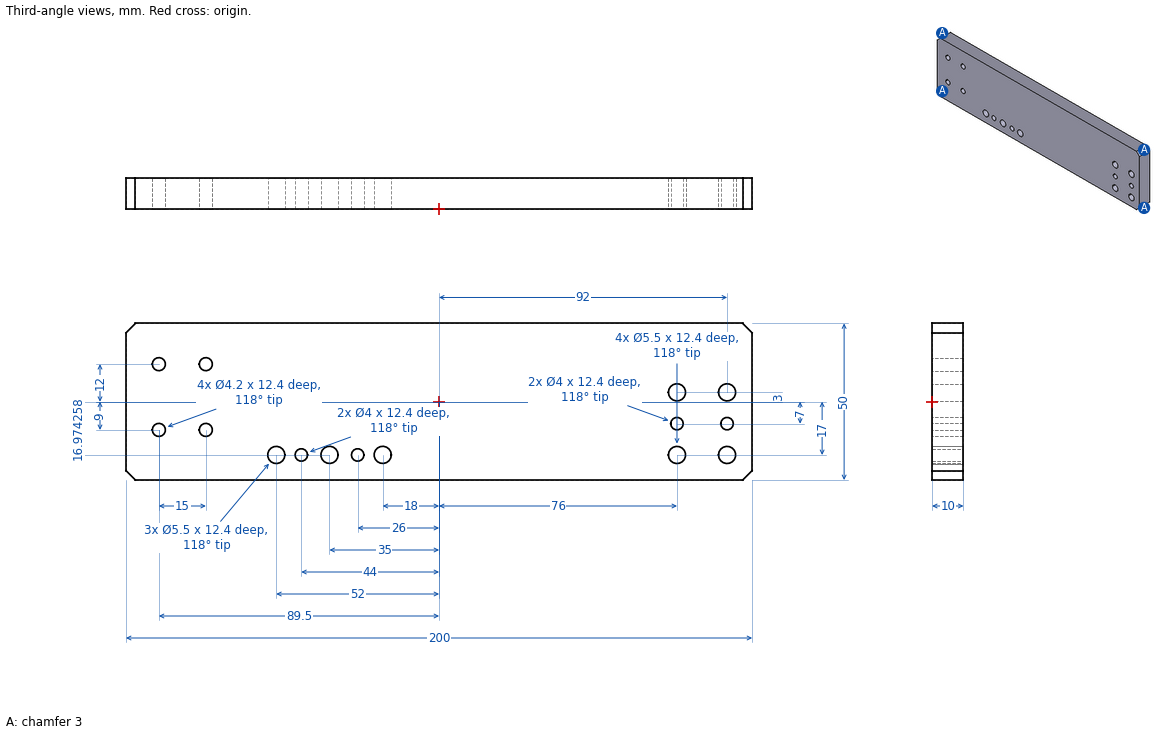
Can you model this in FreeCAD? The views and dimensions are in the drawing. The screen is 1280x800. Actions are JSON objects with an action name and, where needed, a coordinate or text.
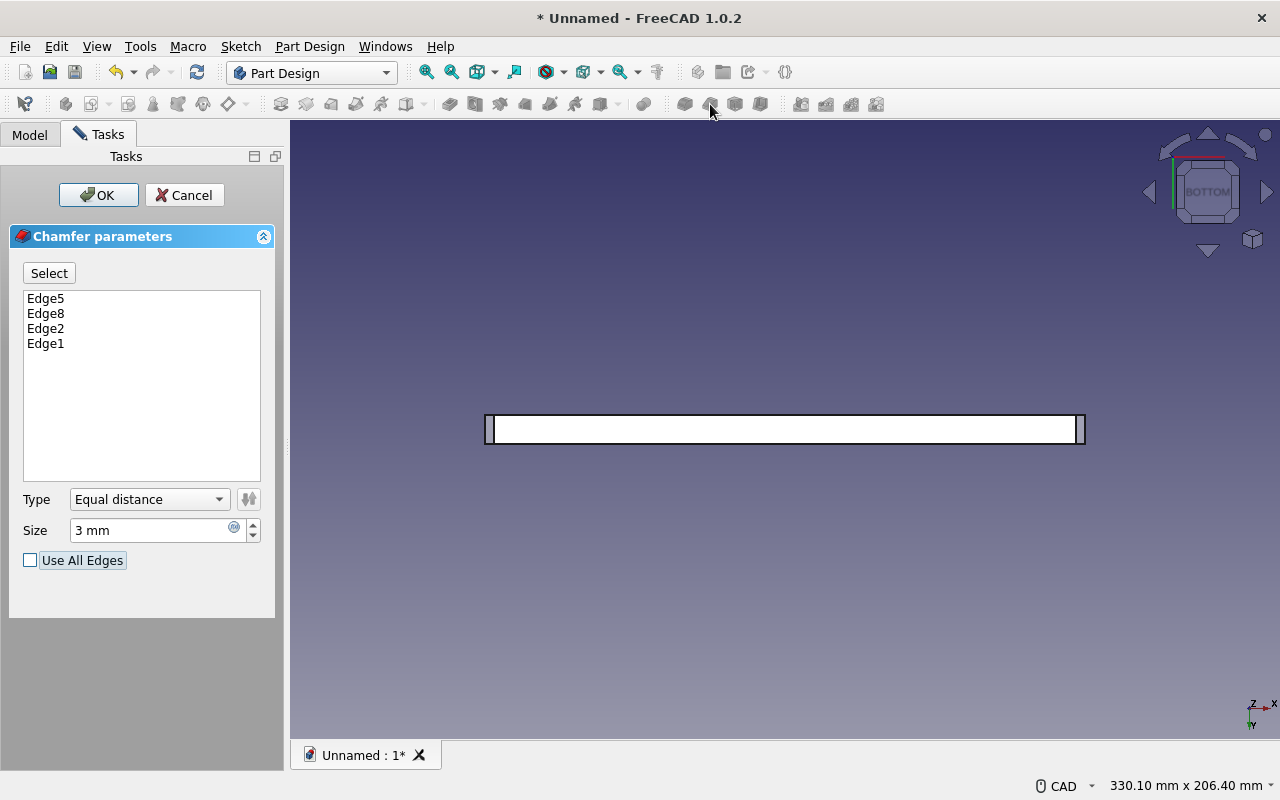
{"action": "left_click", "coordinate": [99, 195]}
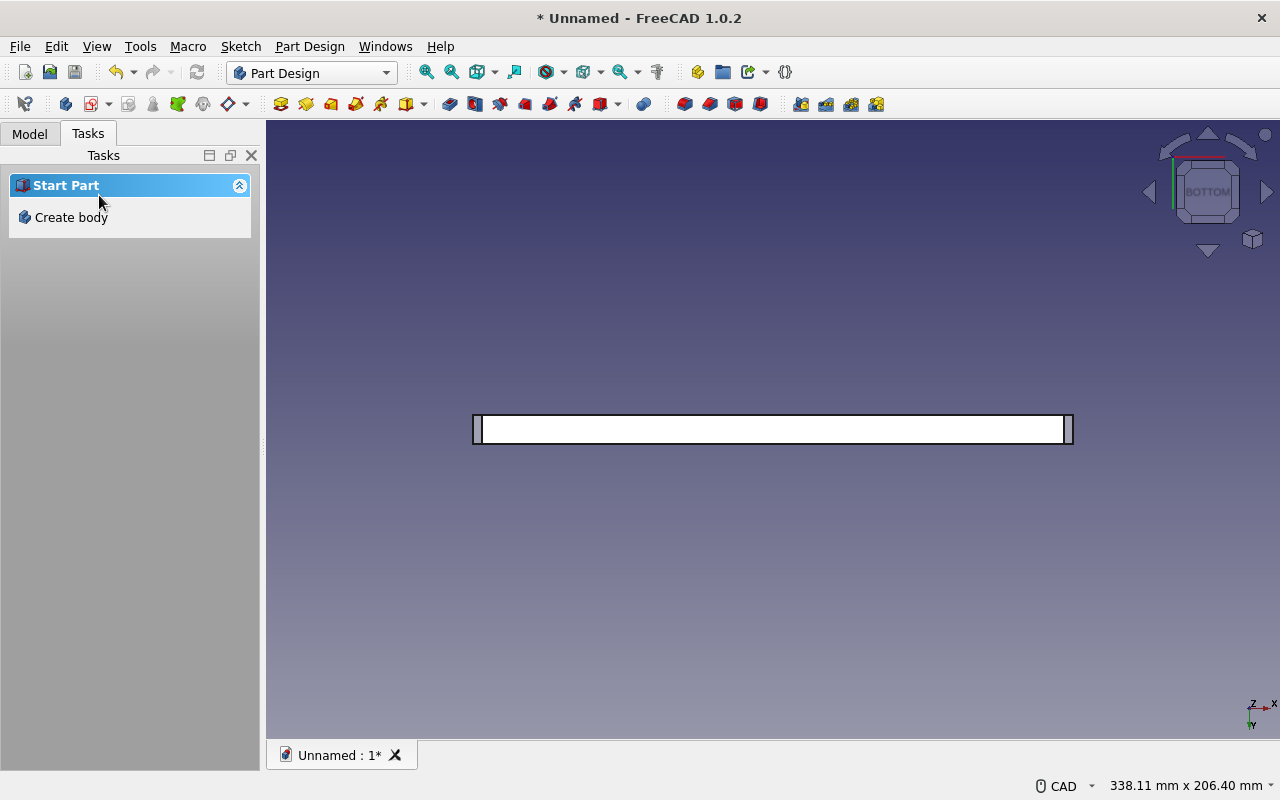
{"action": "key", "text": "4"}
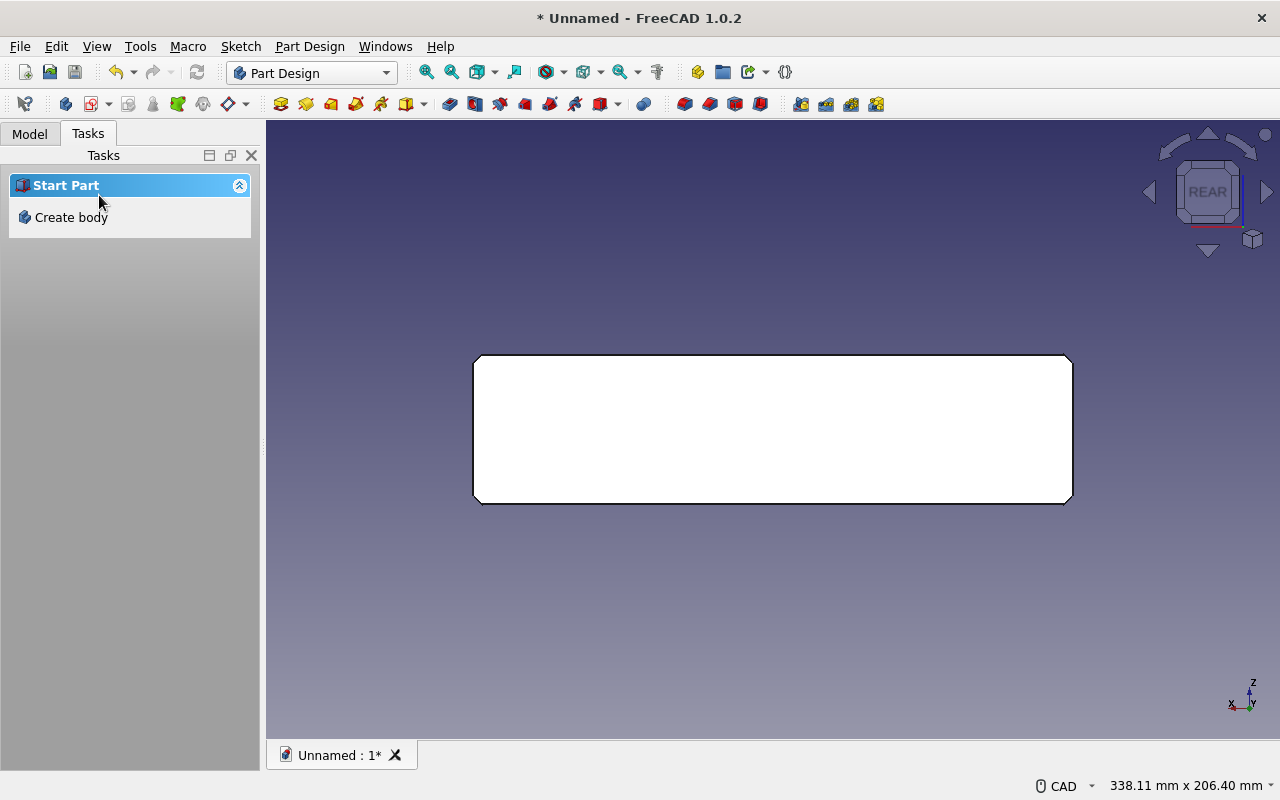
{"action": "left_click", "coordinate": [602, 429]}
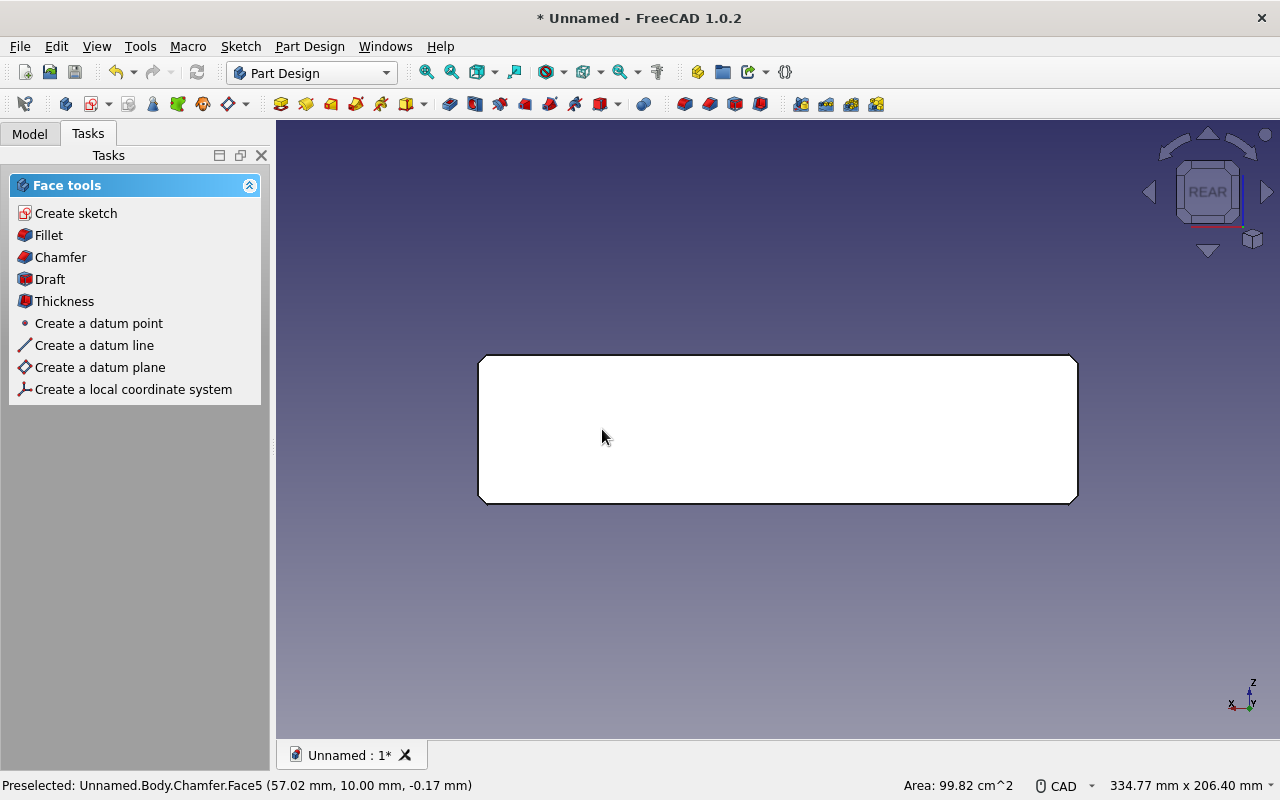
{"action": "left_click", "coordinate": [90, 104]}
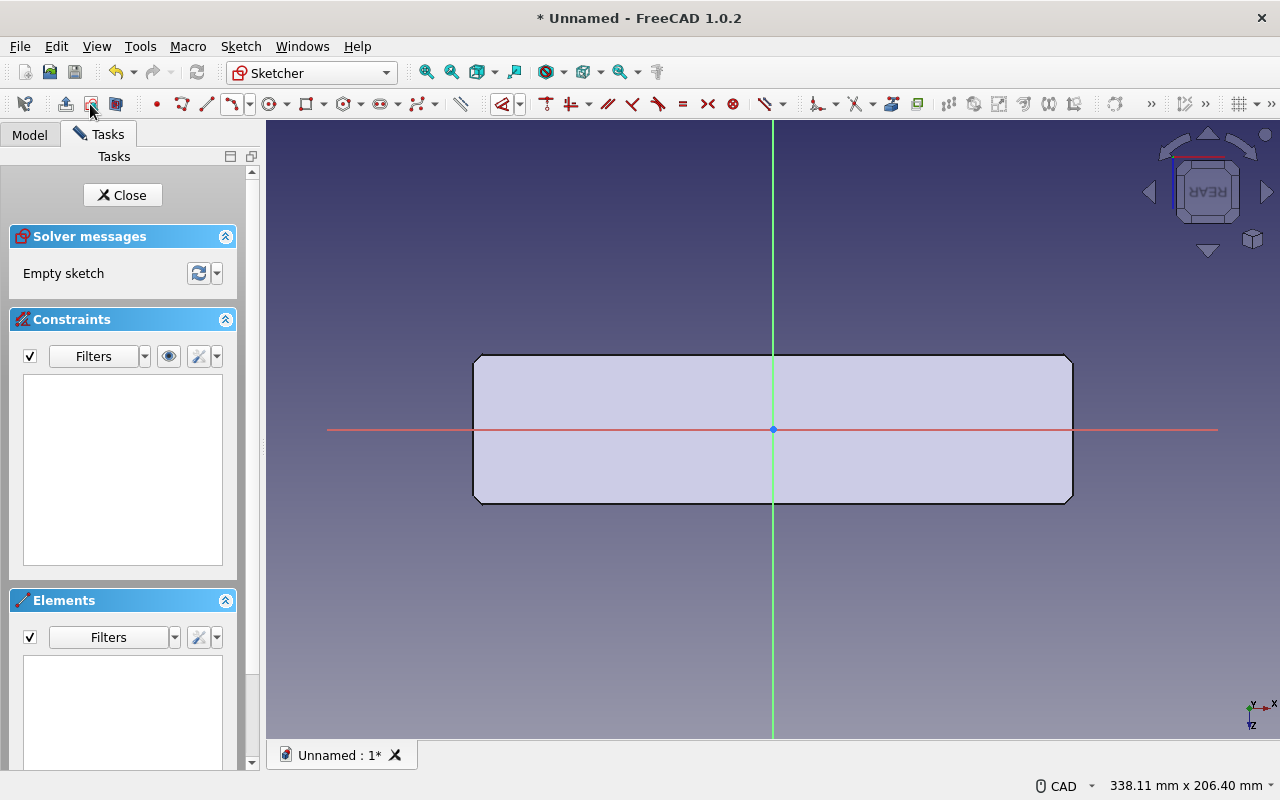
{"action": "scroll", "coordinate": [1106, 403], "scroll_direction": "up", "scroll_amount": 8}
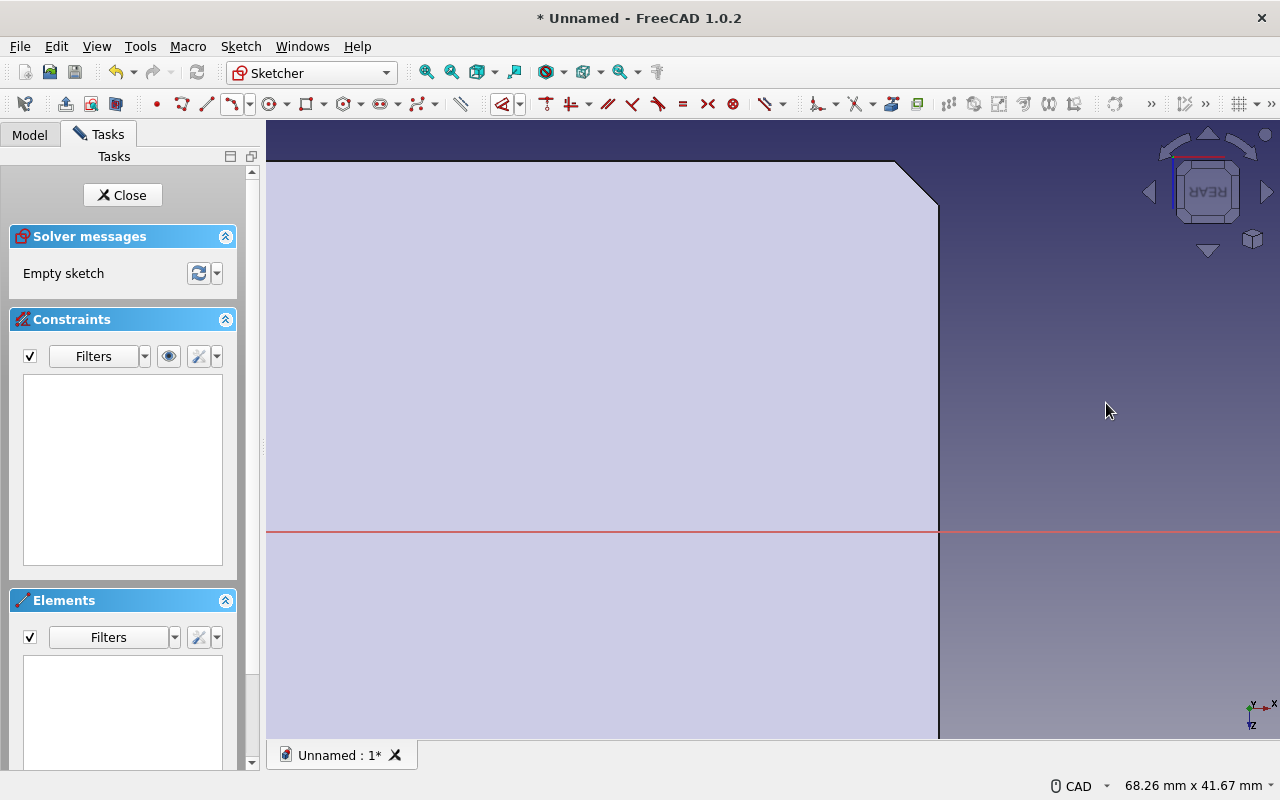
{"action": "key", "text": "g c"}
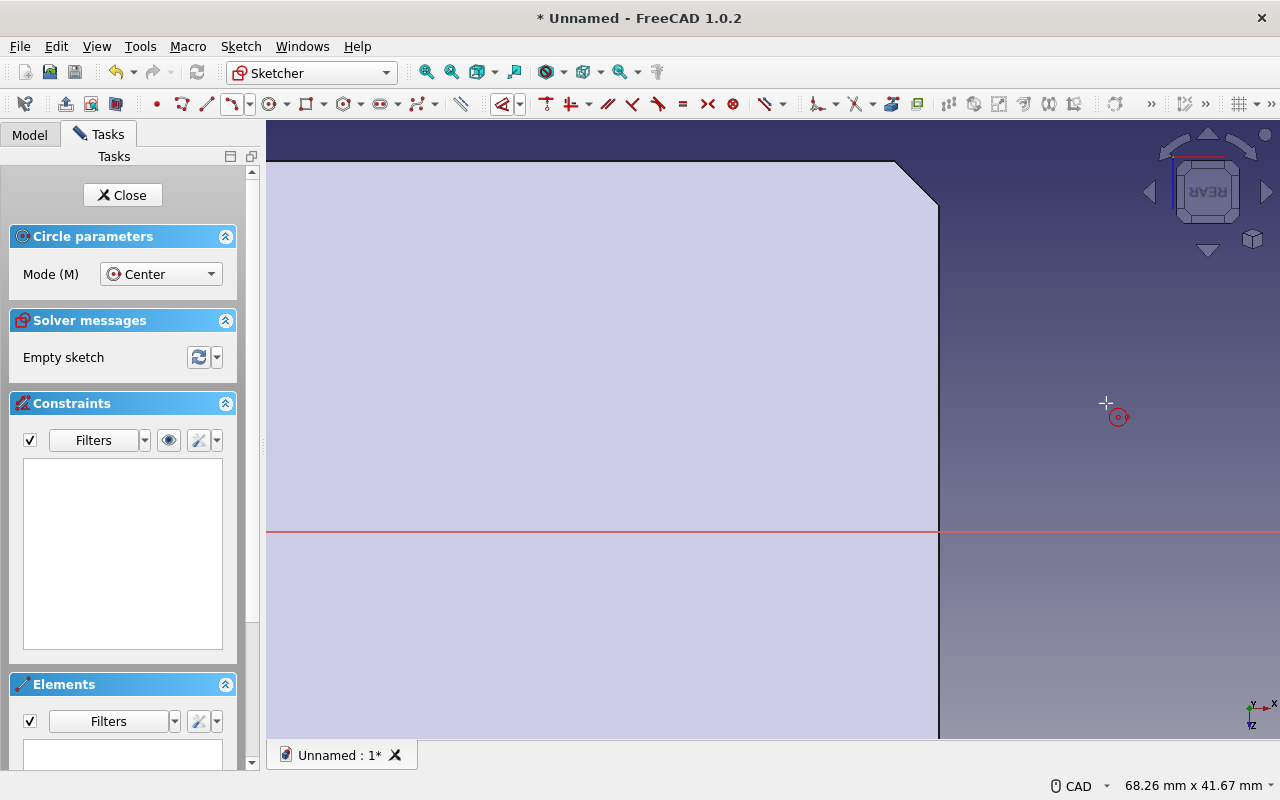
{"action": "left_click", "coordinate": [582, 280]}
{"action": "left_click", "coordinate": [611, 251]}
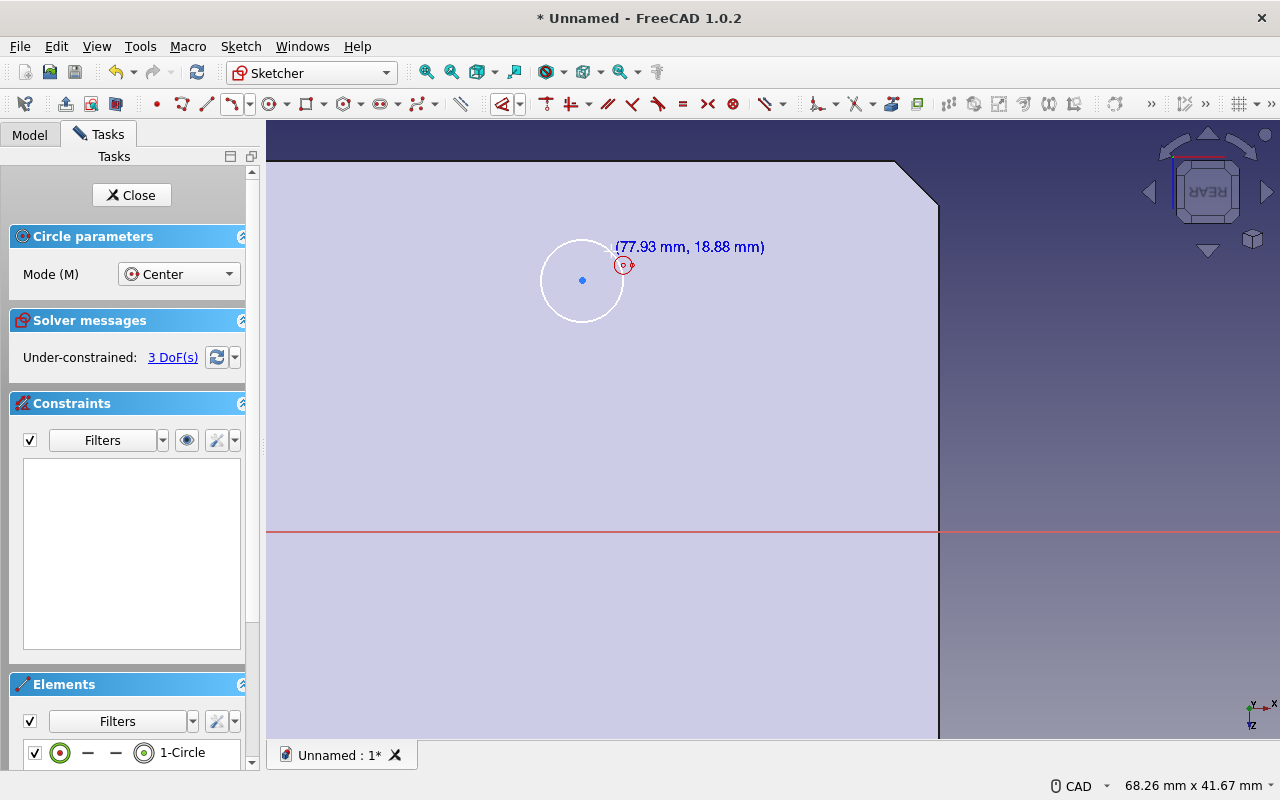
{"action": "left_click", "coordinate": [582, 577]}
{"action": "left_click", "coordinate": [611, 548]}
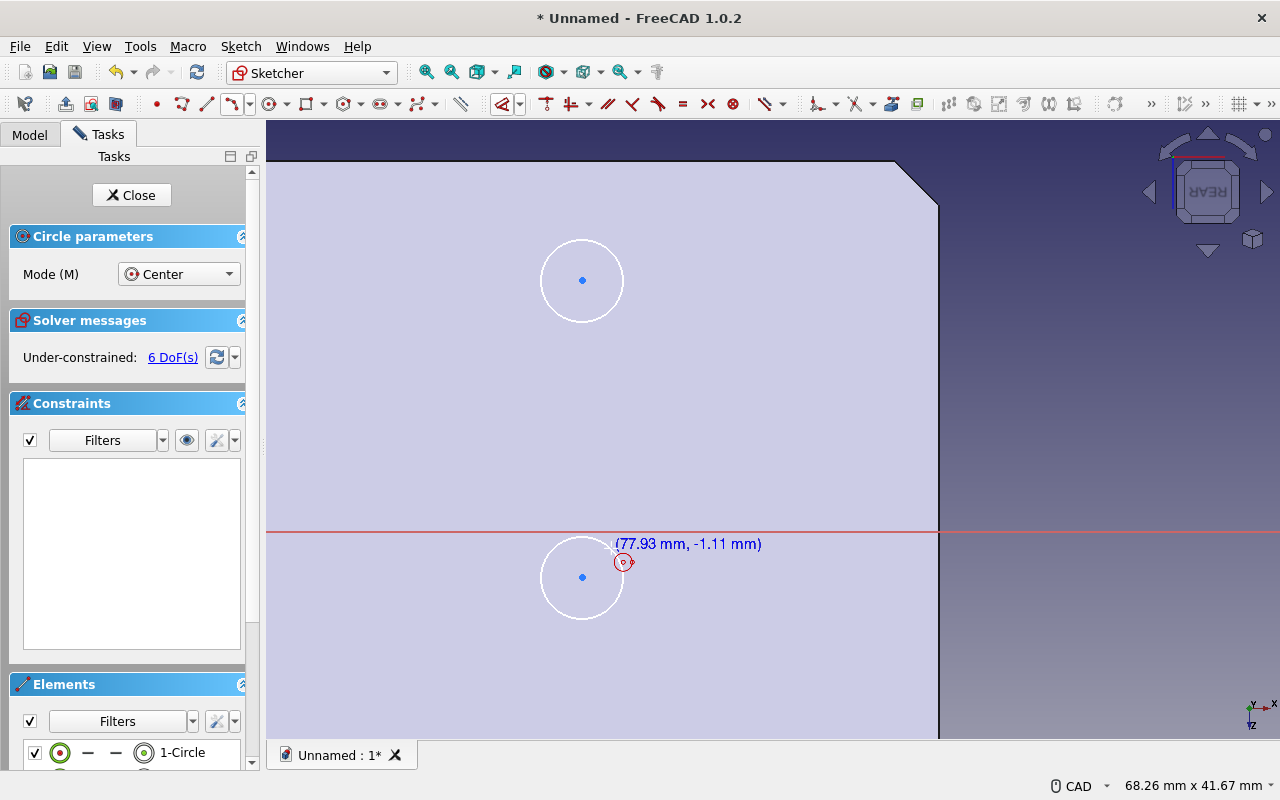
{"action": "left_click", "coordinate": [820, 577]}
{"action": "left_click", "coordinate": [849, 548]}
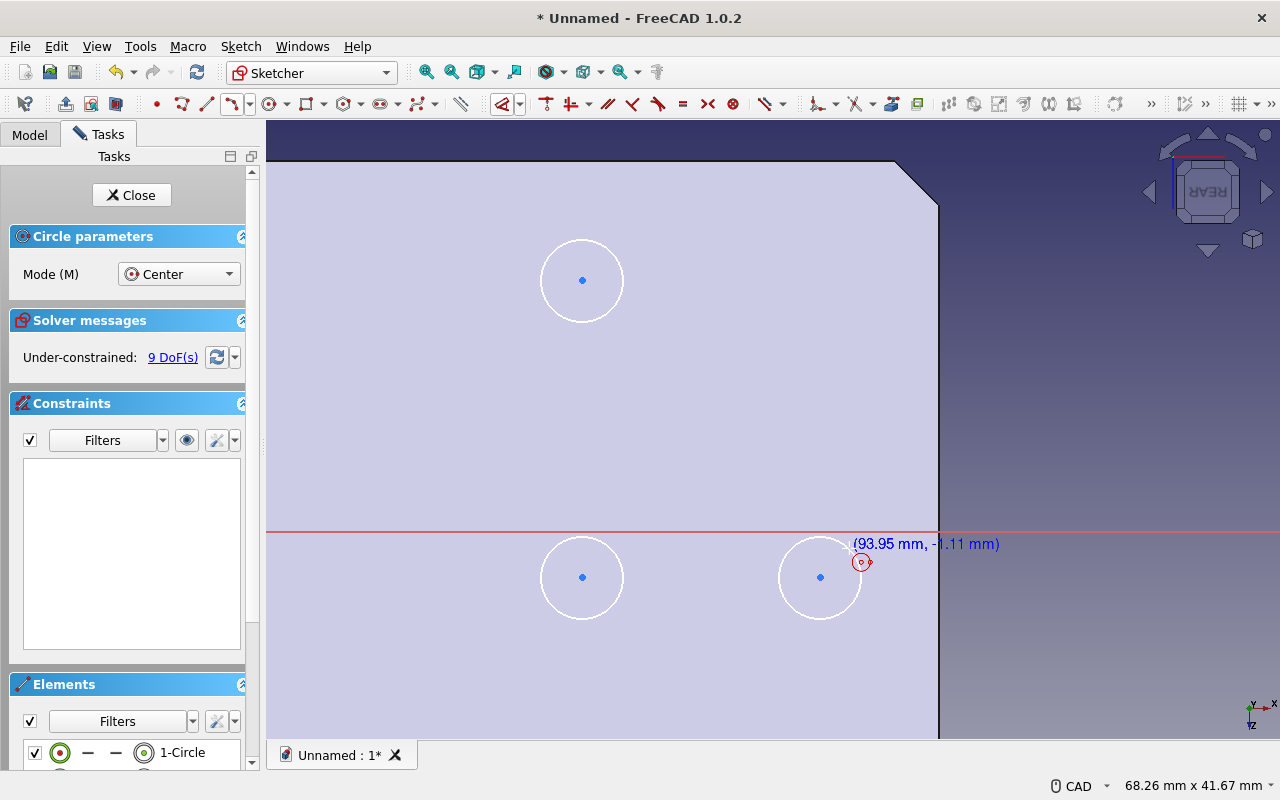
{"action": "left_click", "coordinate": [820, 280]}
{"action": "left_click", "coordinate": [849, 251]}
{"action": "key", "text": "Escape"}